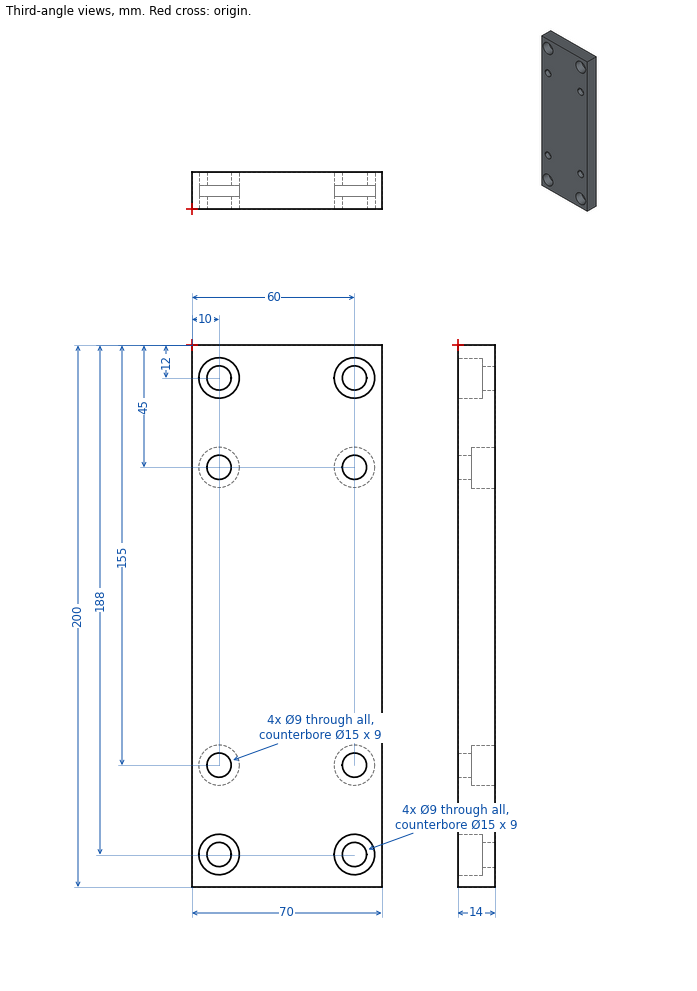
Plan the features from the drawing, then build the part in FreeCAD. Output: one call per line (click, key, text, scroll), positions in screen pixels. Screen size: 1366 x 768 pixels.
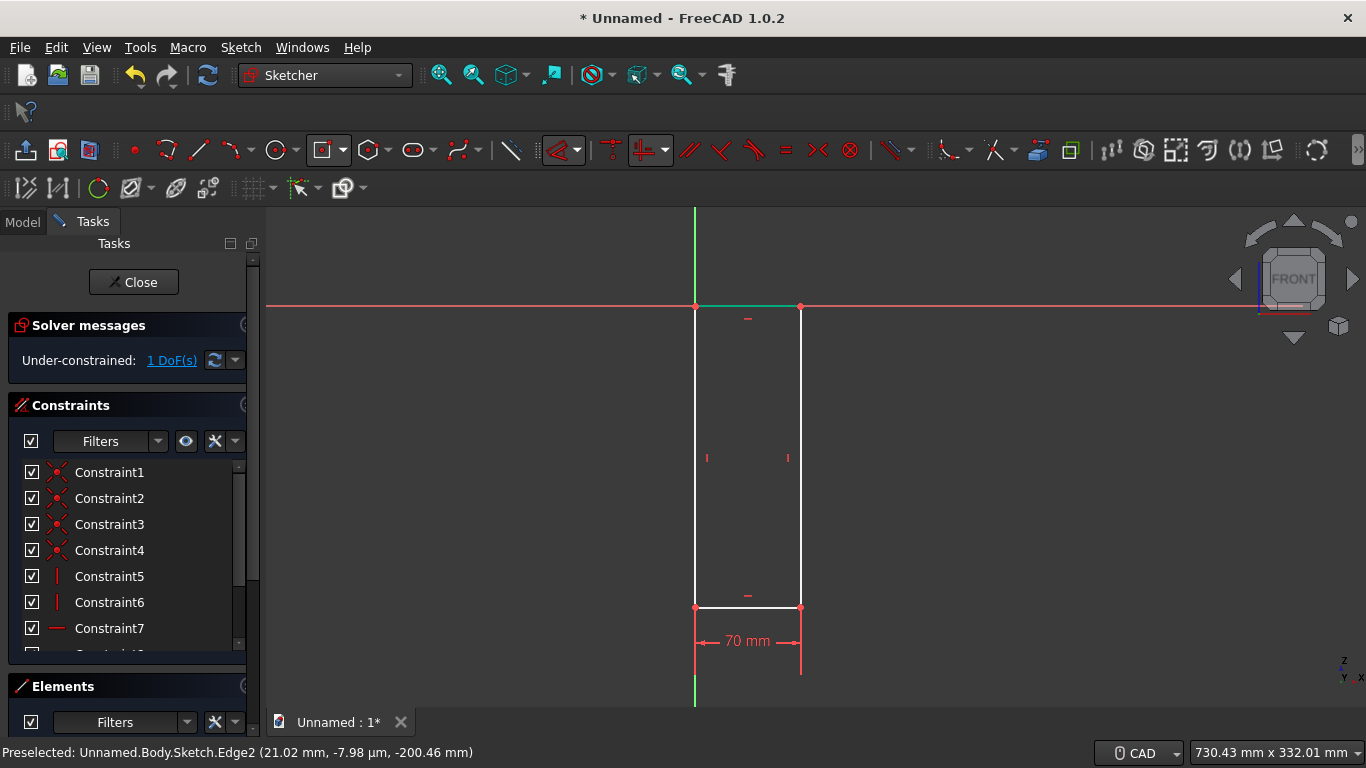
click(695, 397)
click(661, 457)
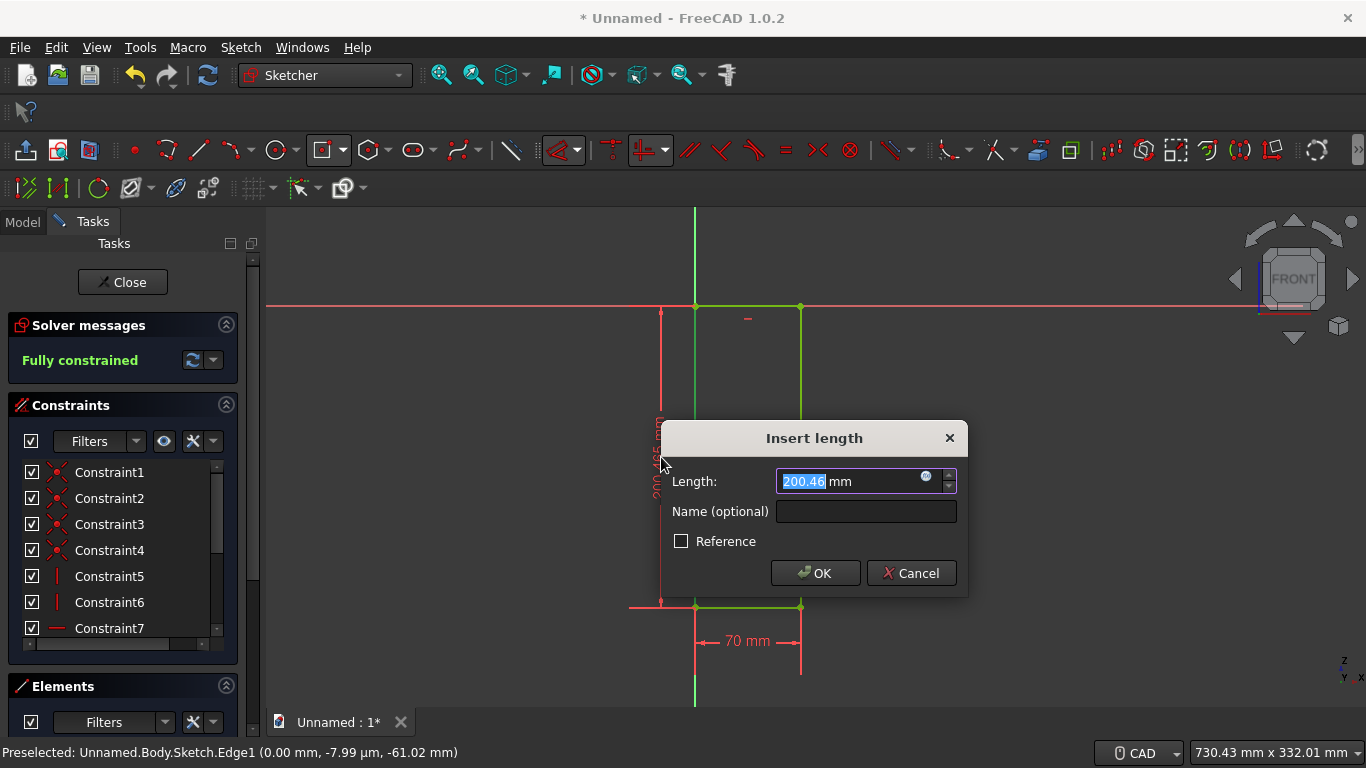
text(200)
key(Return)
key(Escape)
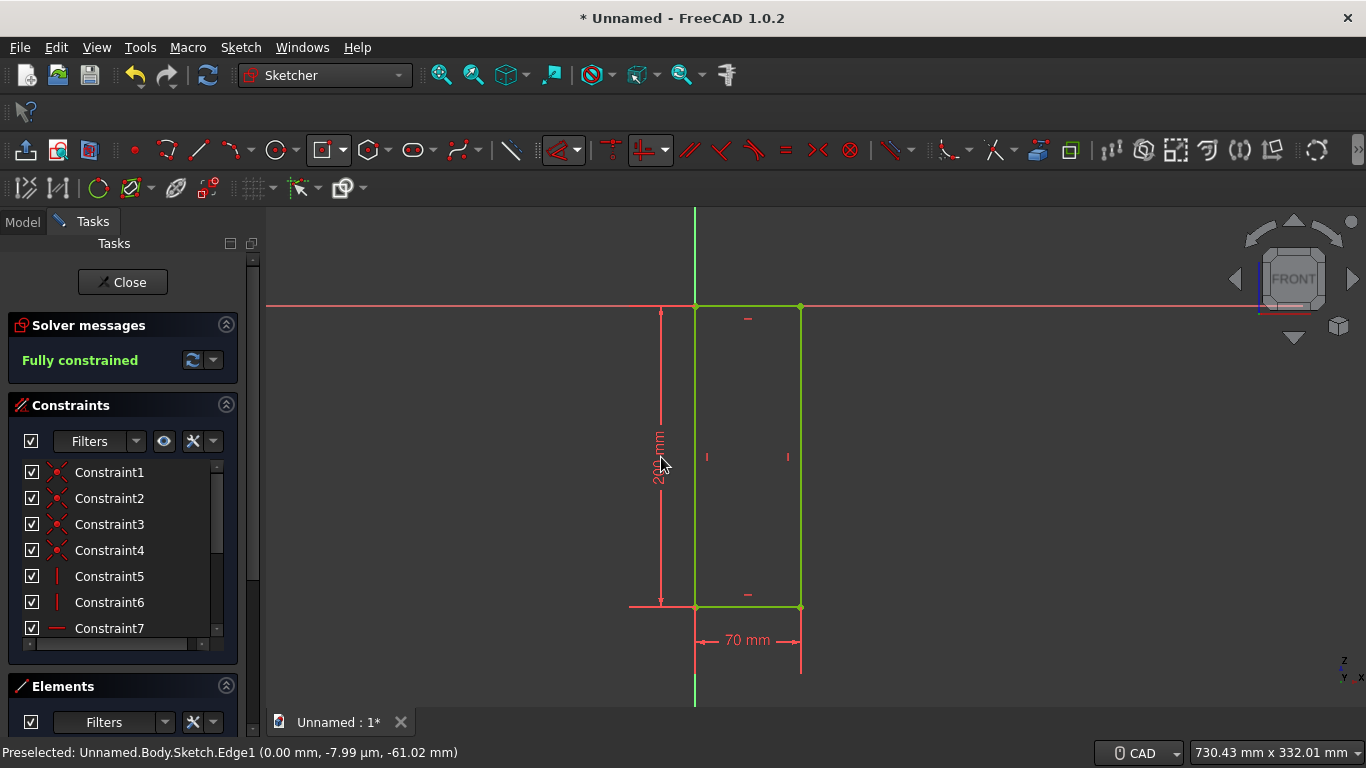
click(123, 282)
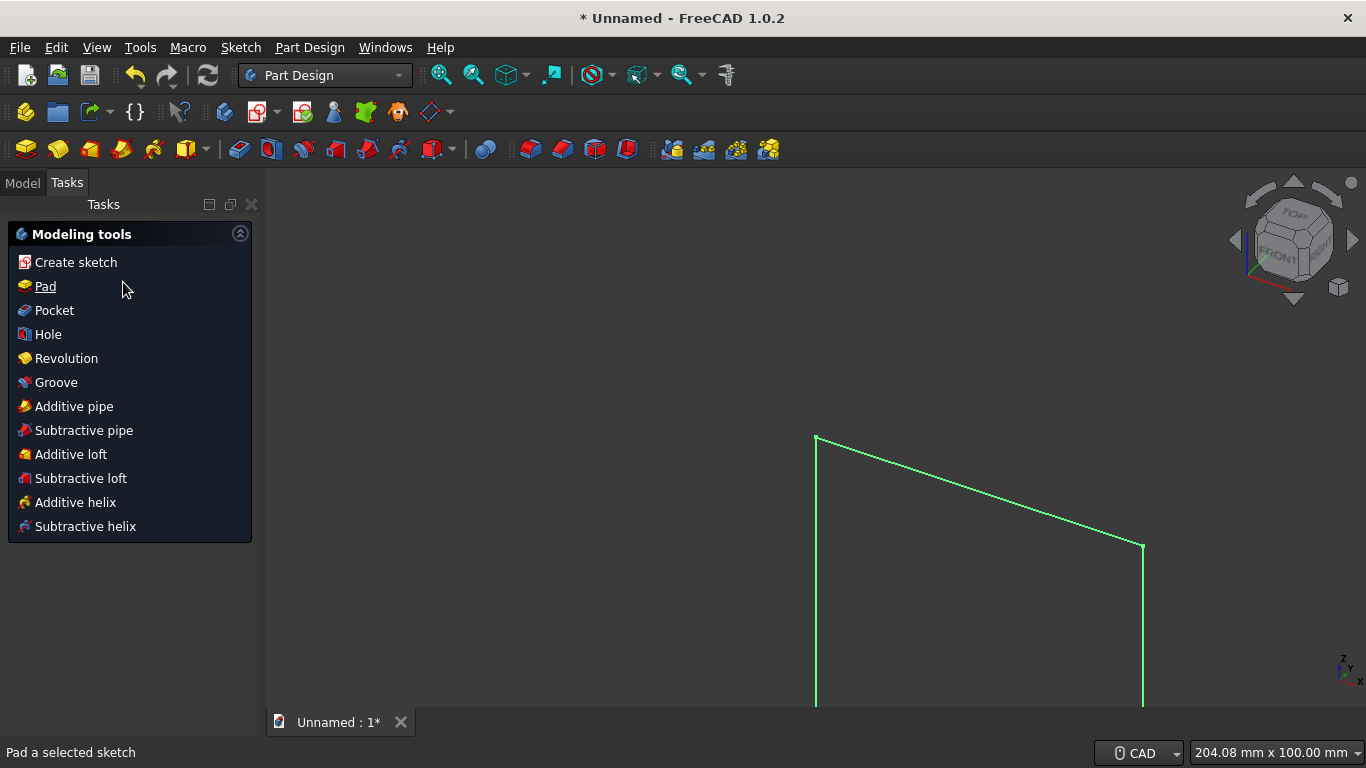
click(26, 150)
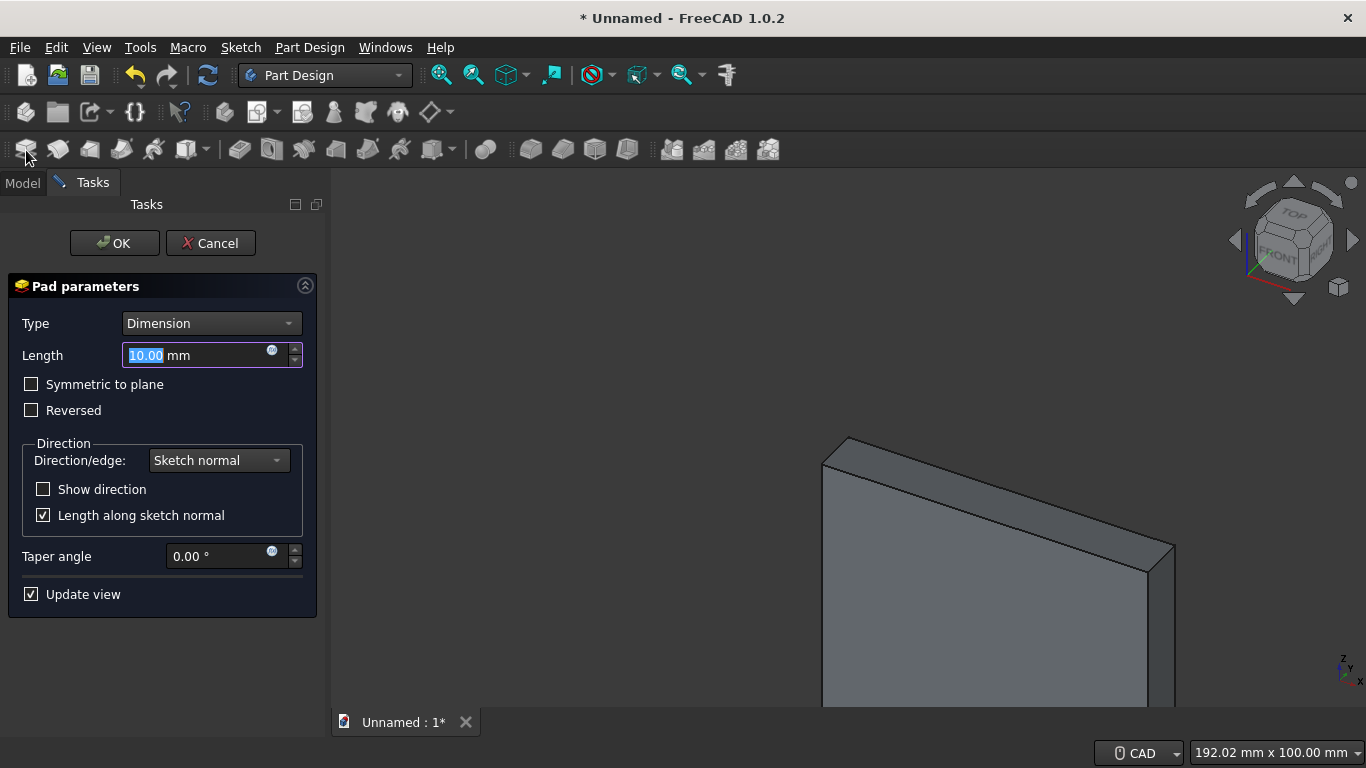
text(14)
key(Tab)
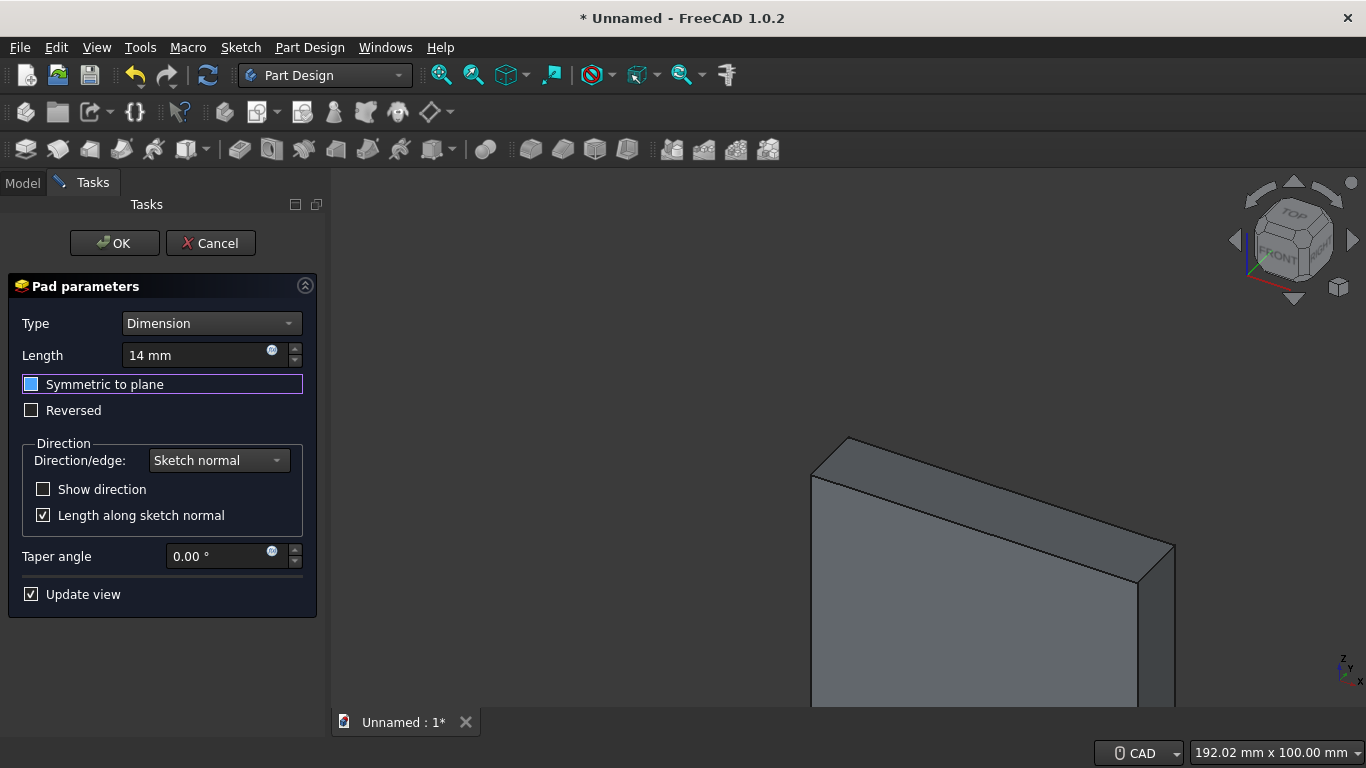
click(30, 410)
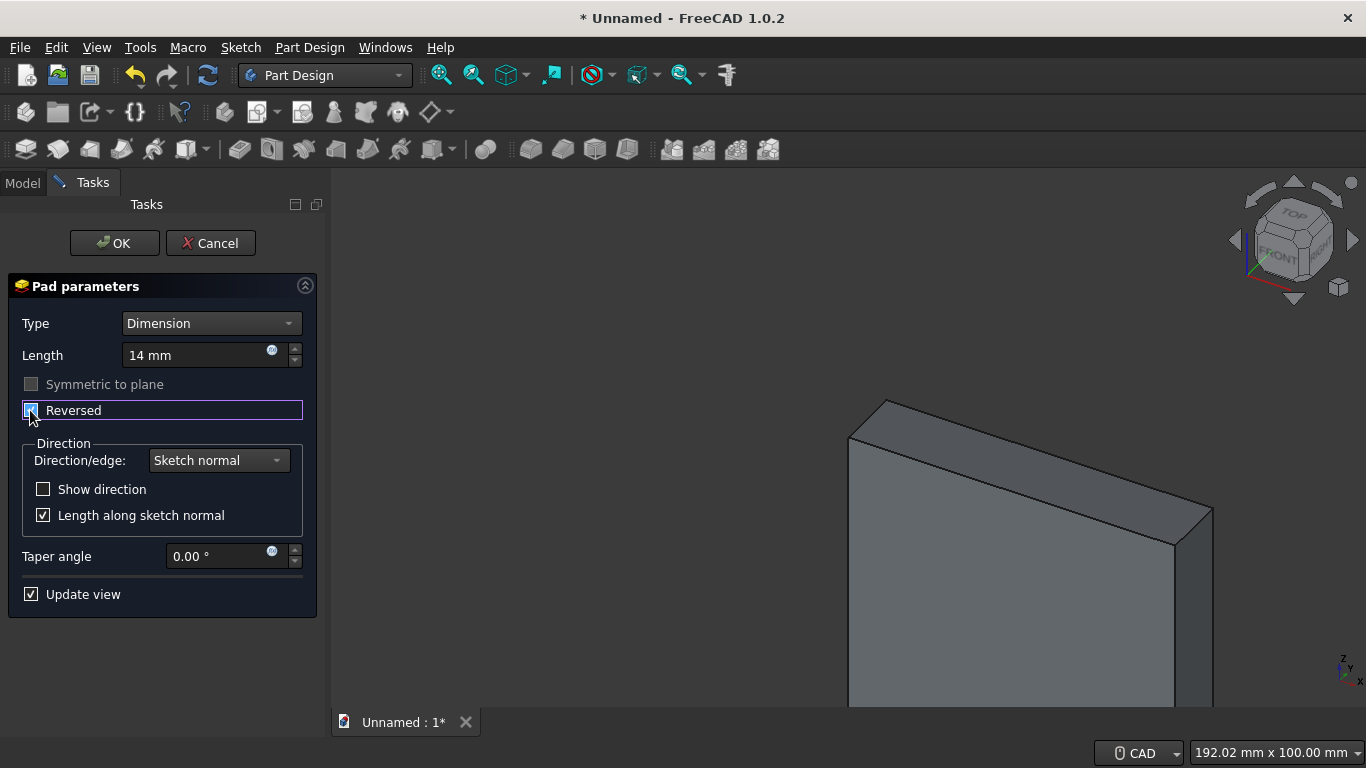
click(115, 243)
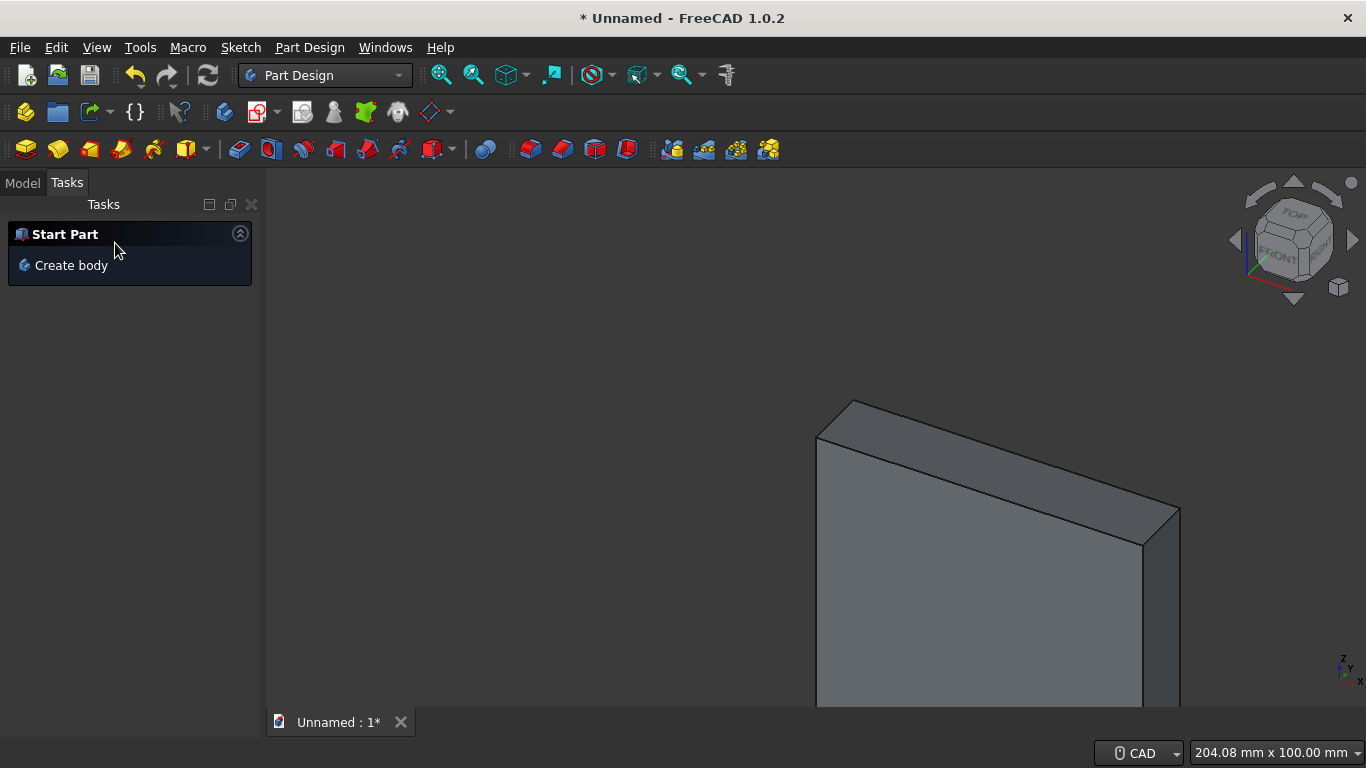
key(v)
key(f)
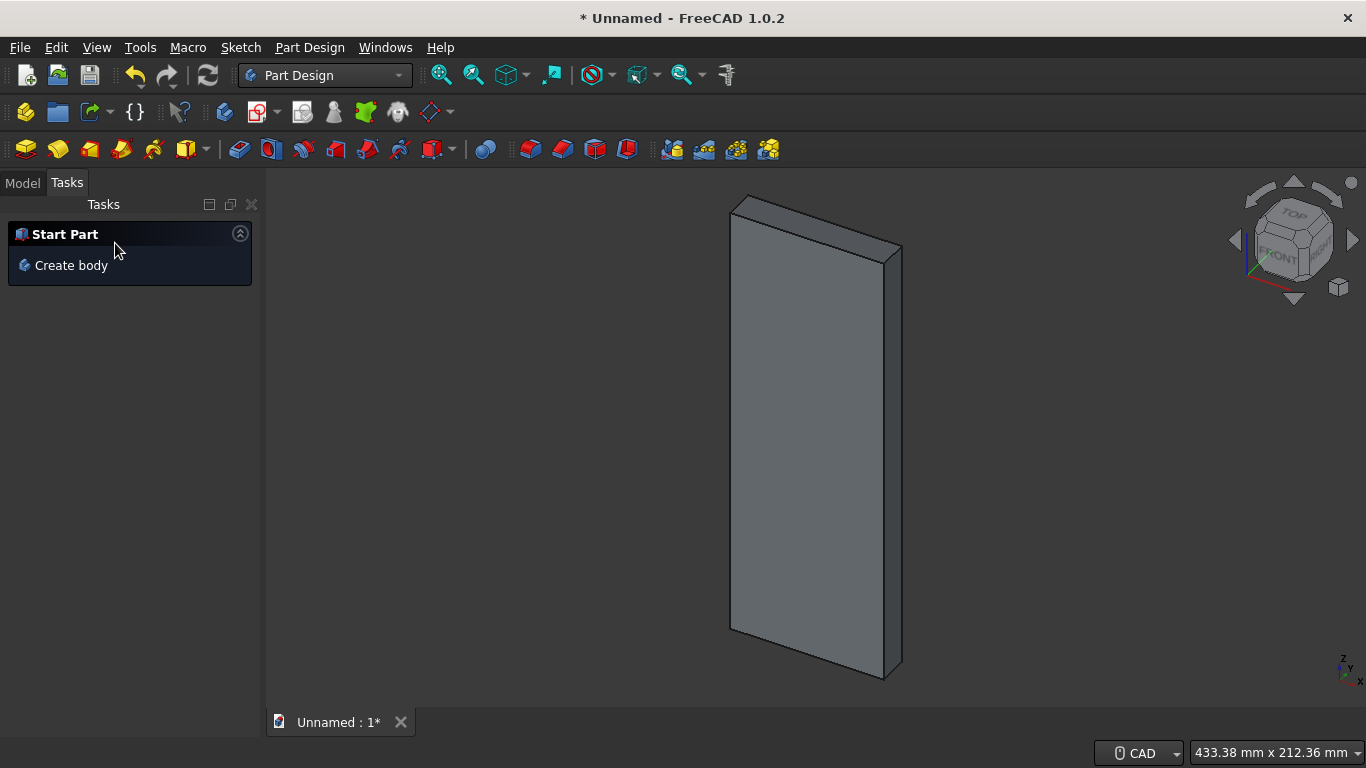
key(4)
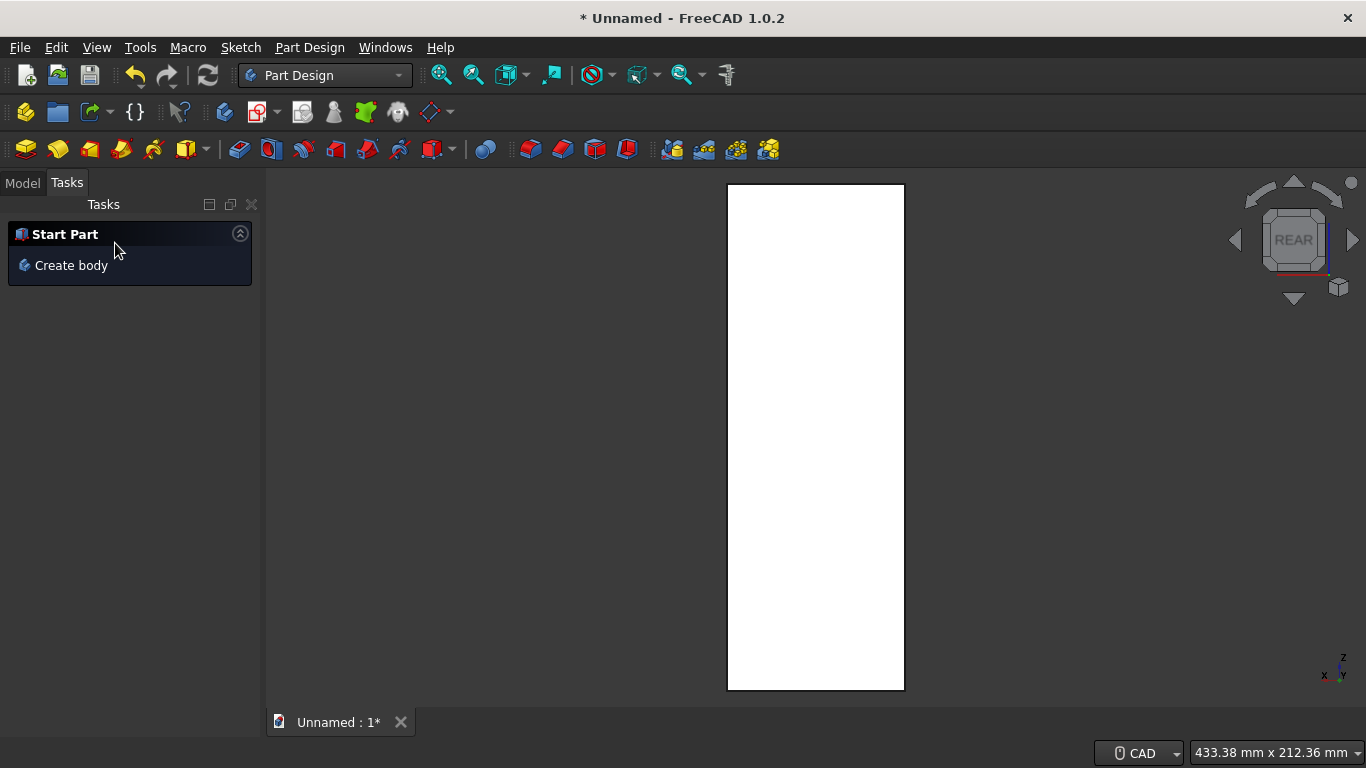
click(816, 291)